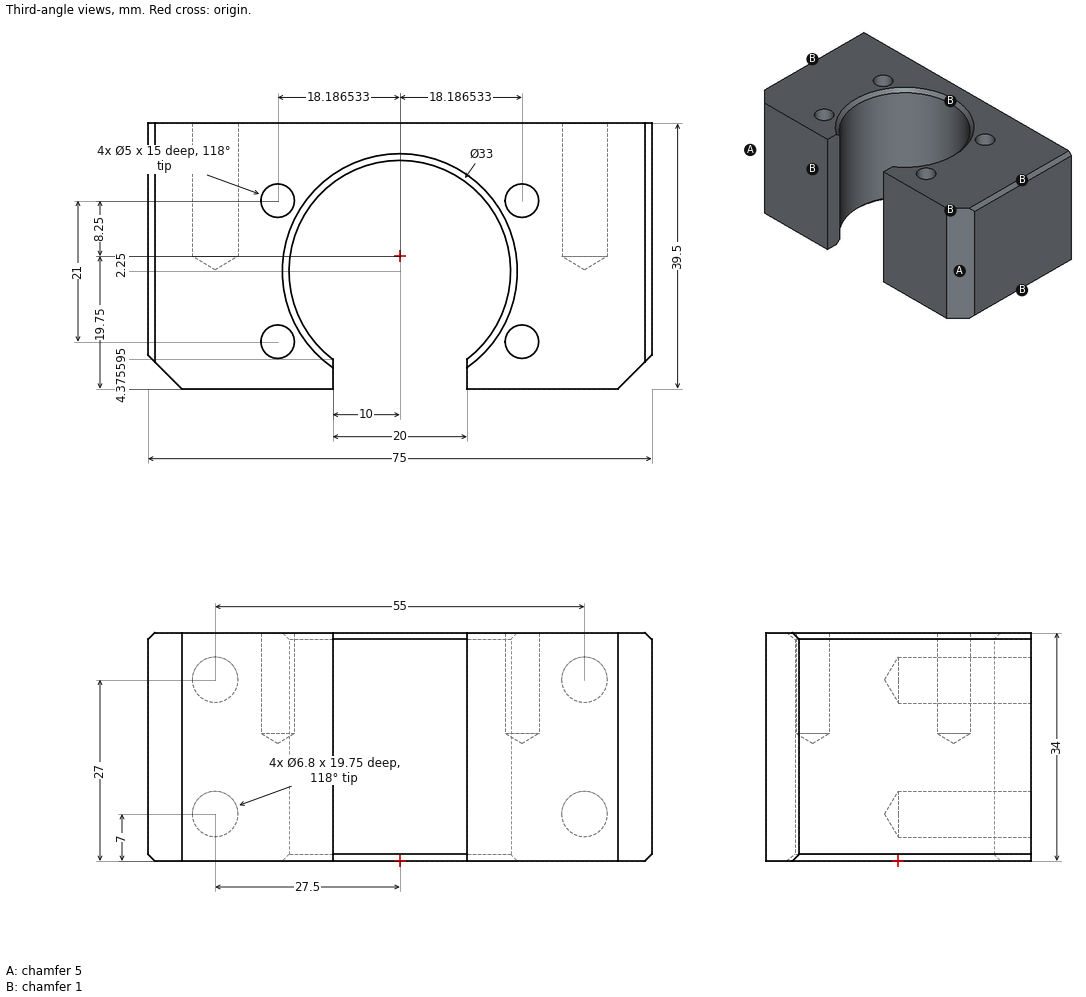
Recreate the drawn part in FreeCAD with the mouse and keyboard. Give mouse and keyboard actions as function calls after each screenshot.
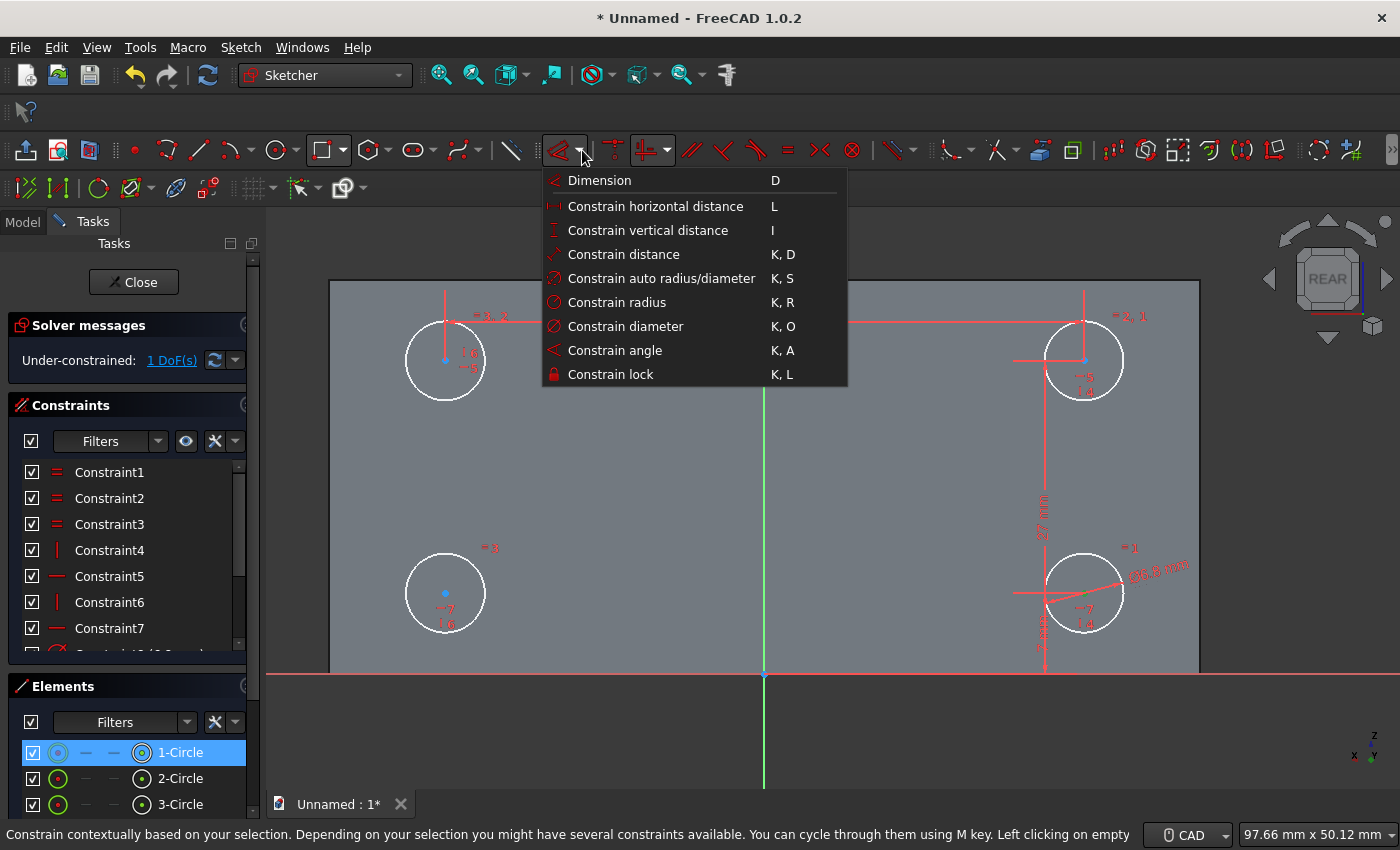
click(695, 206)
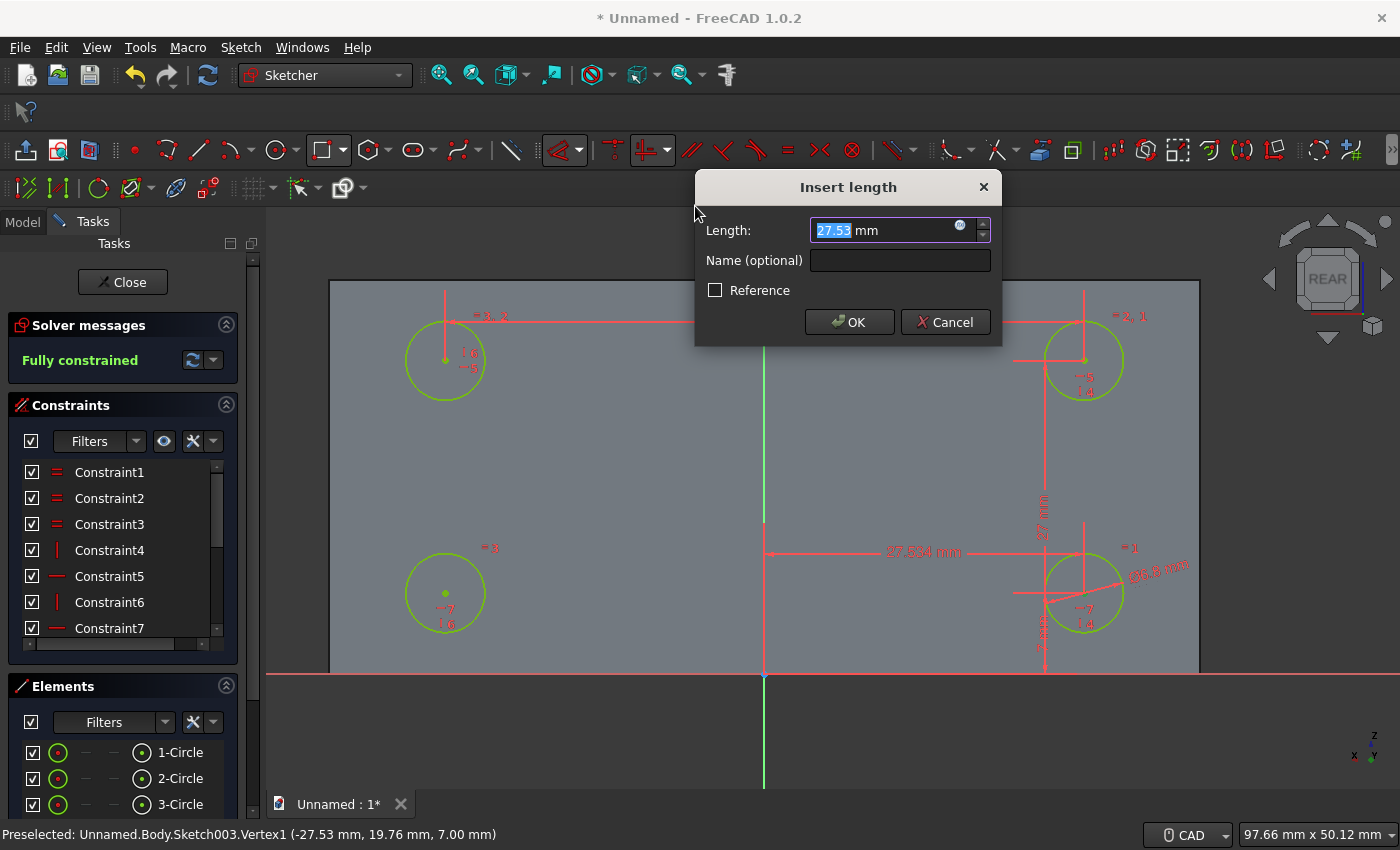
text(27.5)
key(Return)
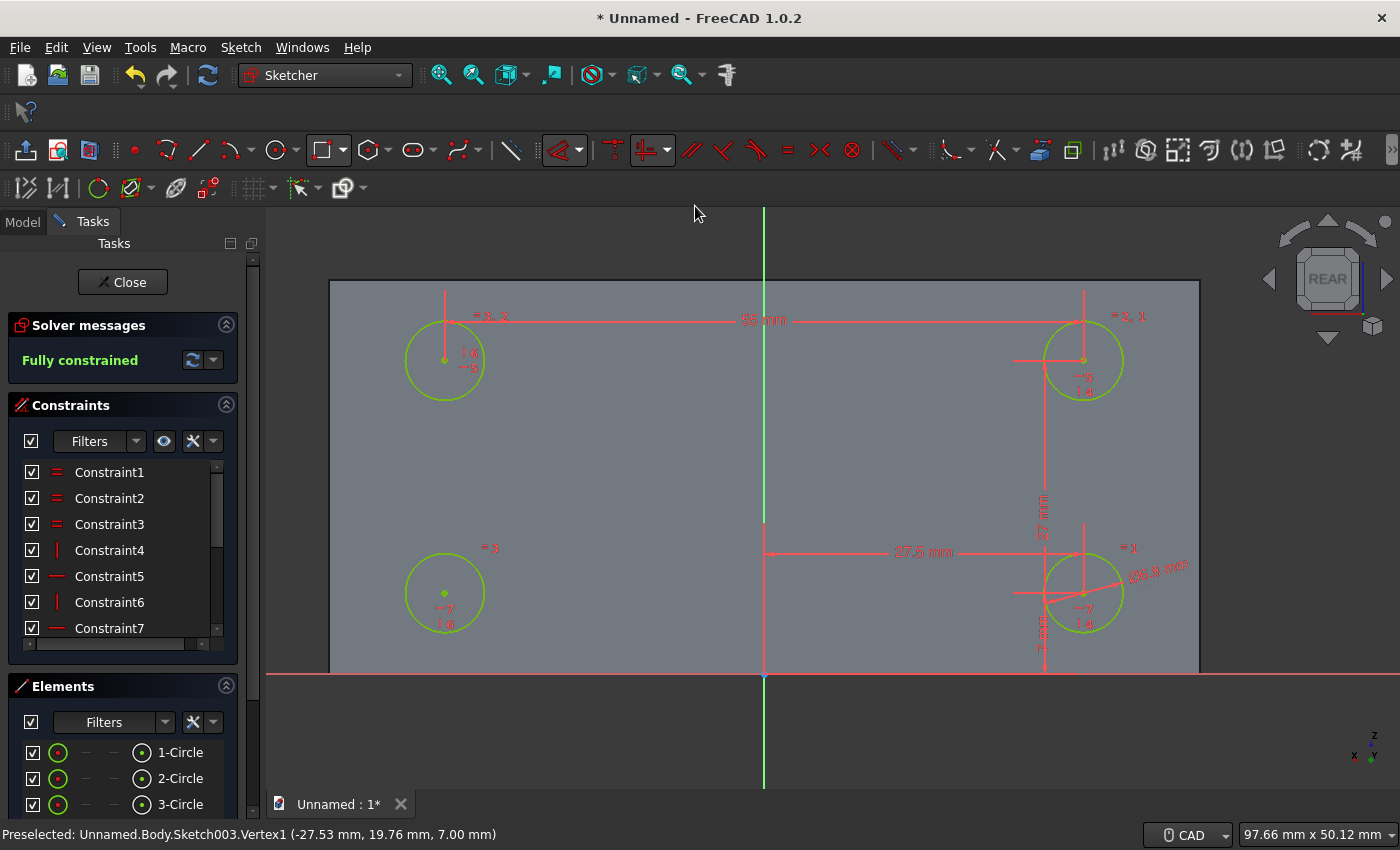
click(123, 282)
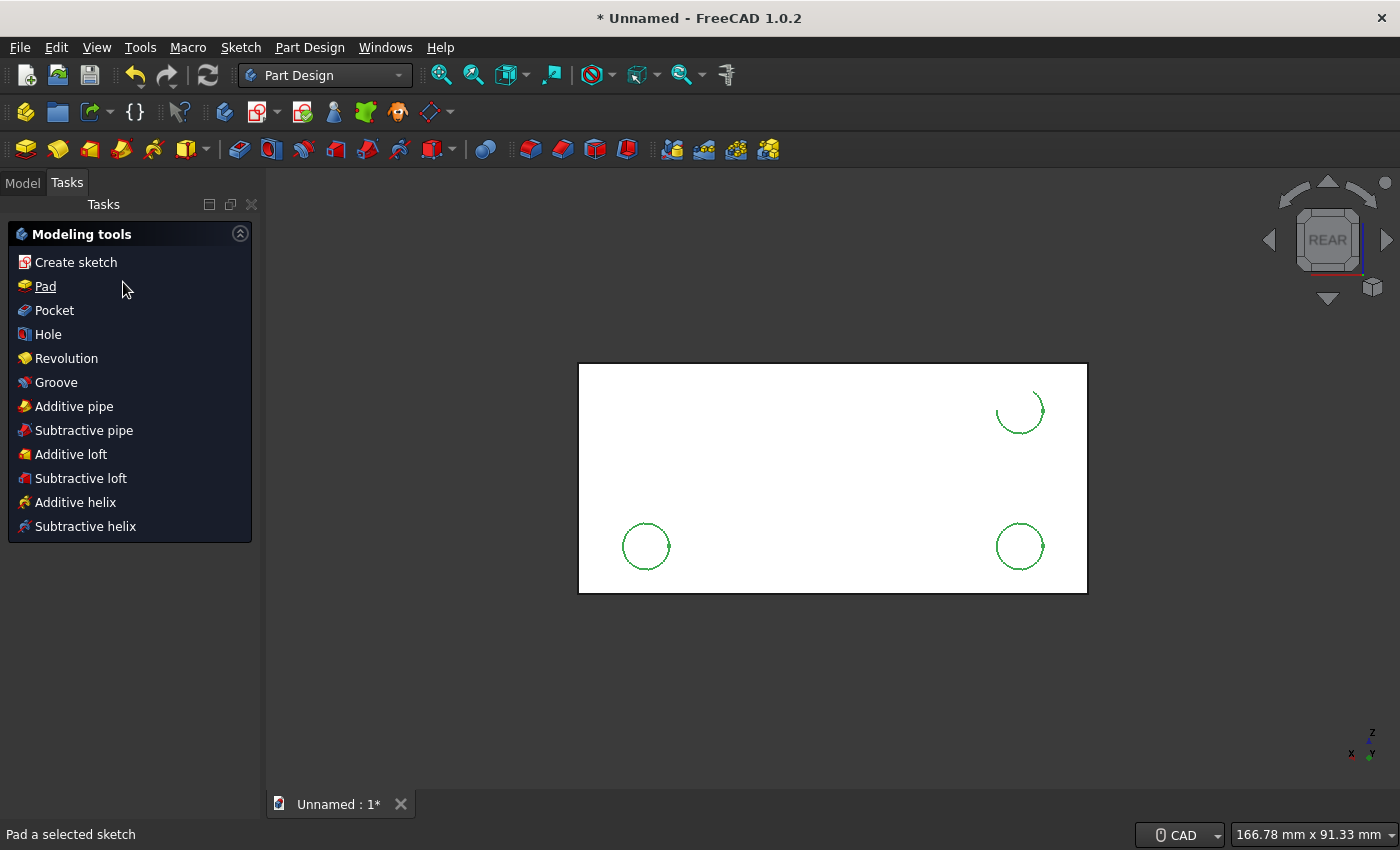
click(272, 150)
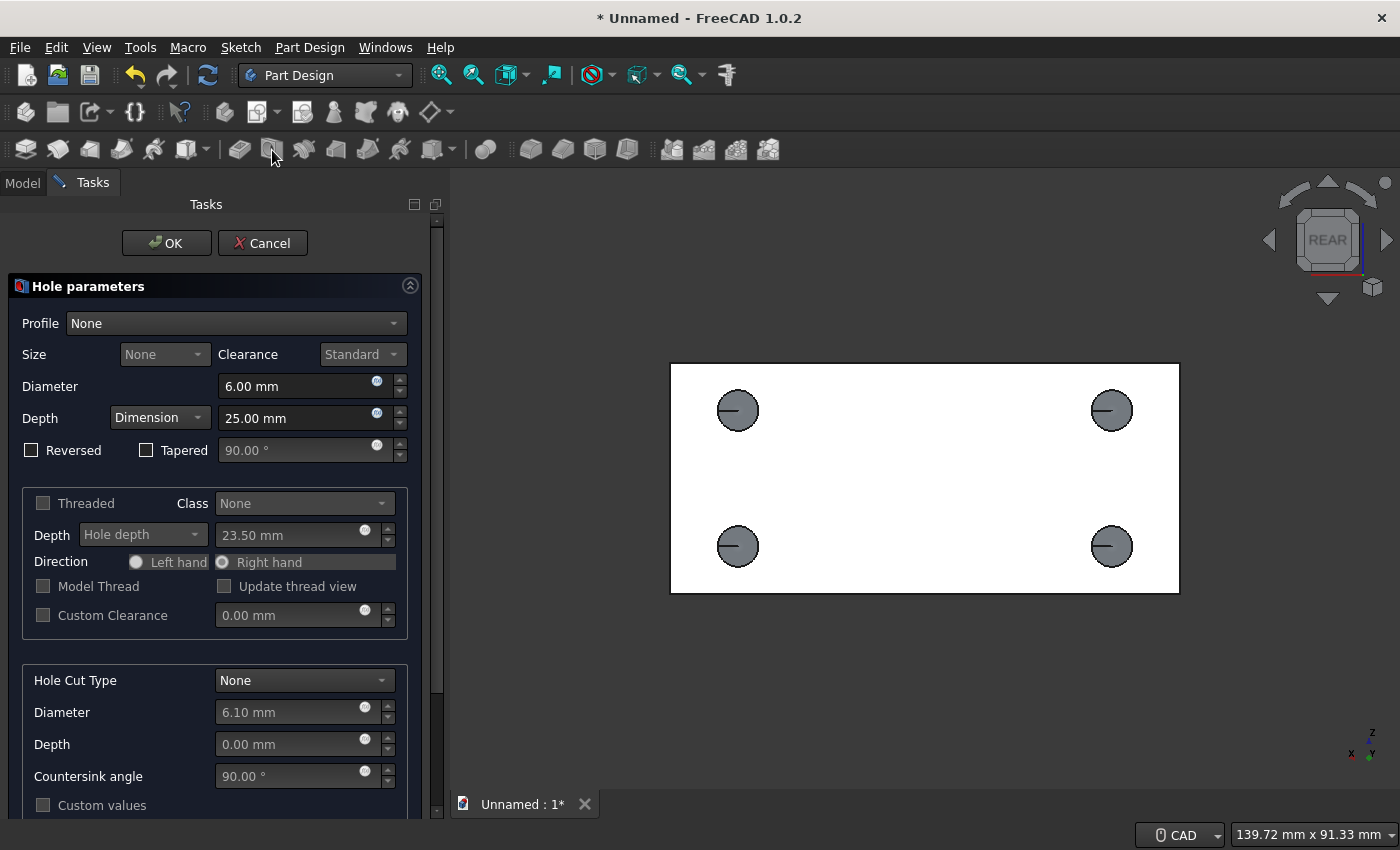
triple_click(305, 386)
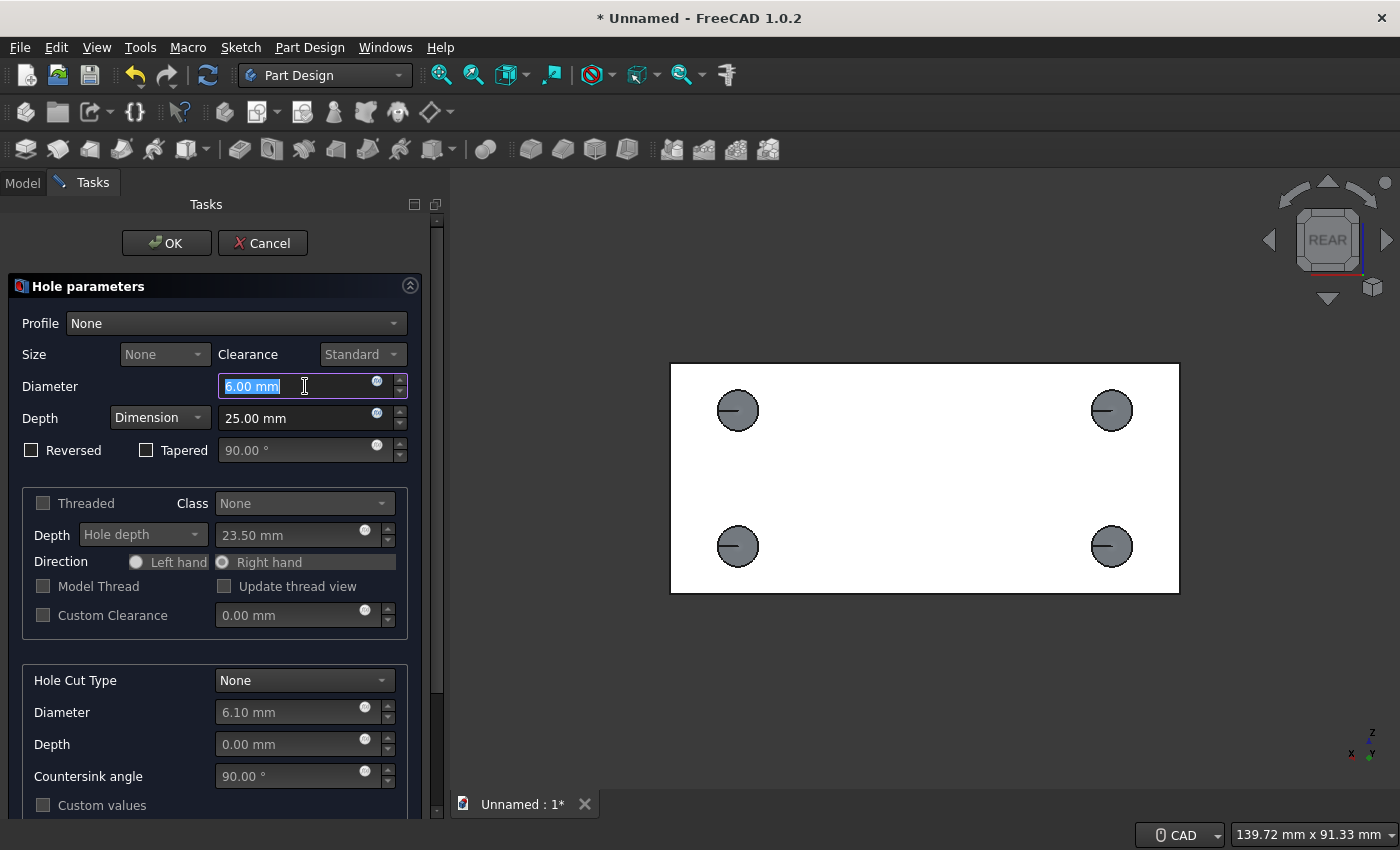
text(6.8)
key(Tab)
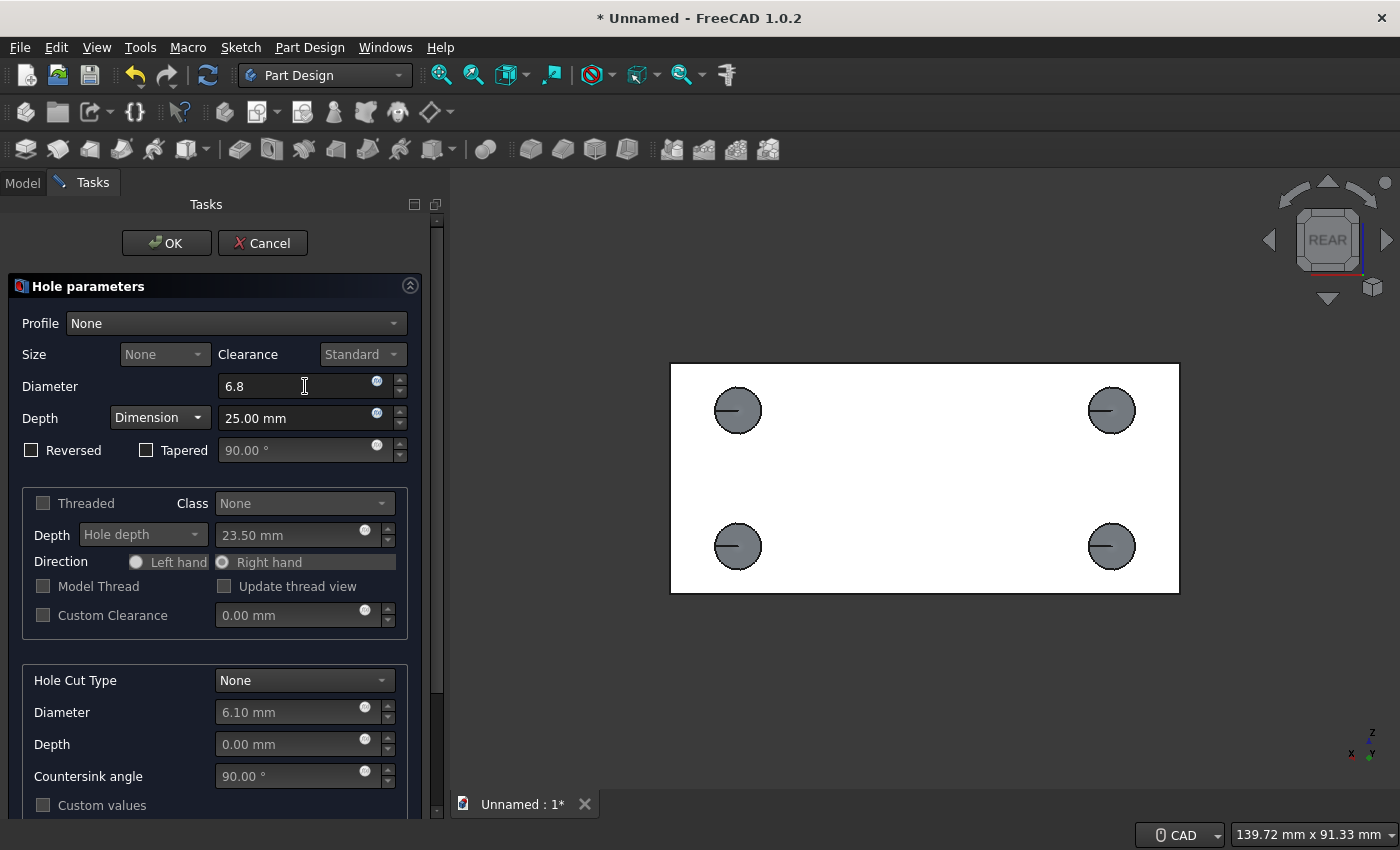
triple_click(305, 418)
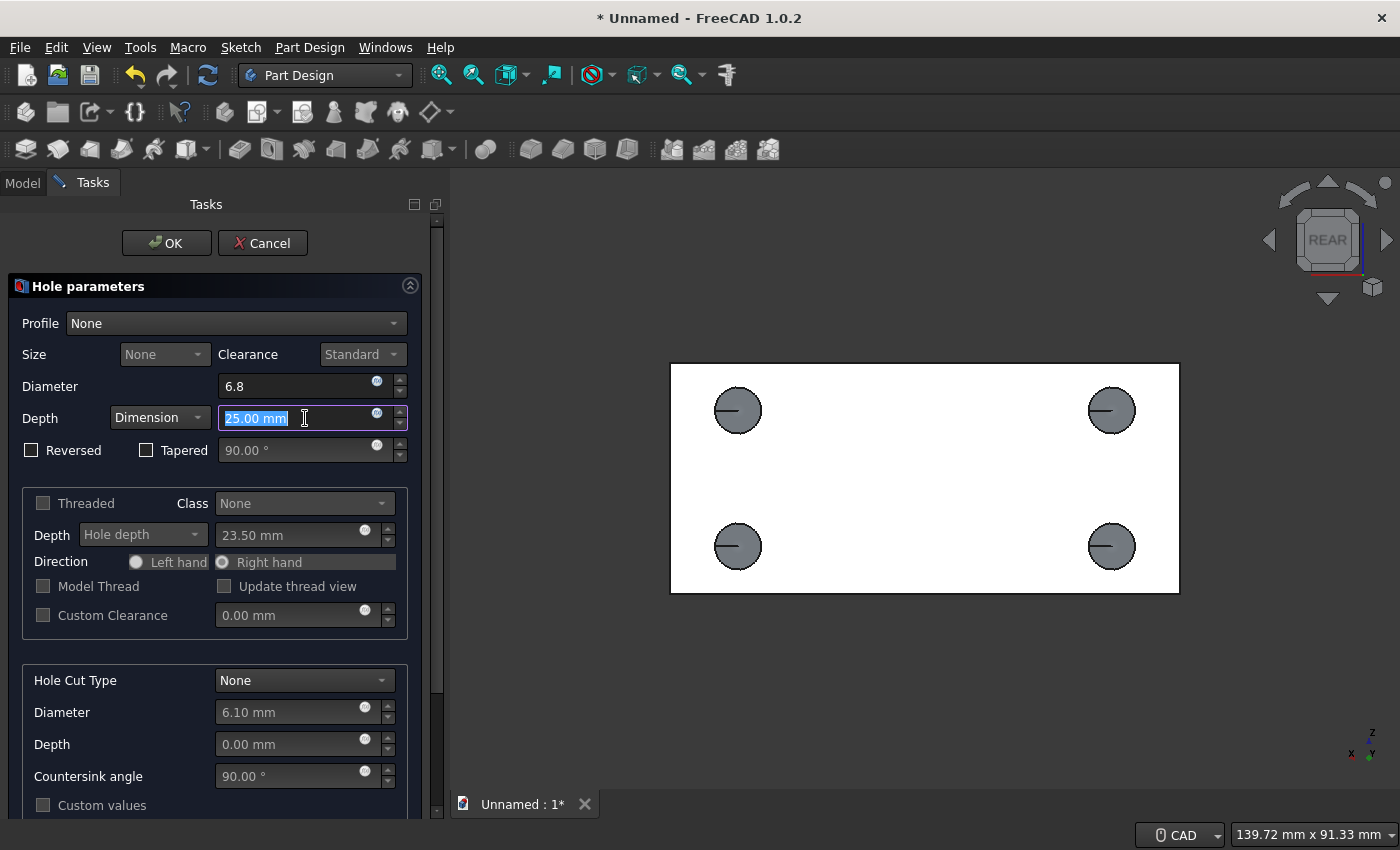
text(19.75)
key(Tab)